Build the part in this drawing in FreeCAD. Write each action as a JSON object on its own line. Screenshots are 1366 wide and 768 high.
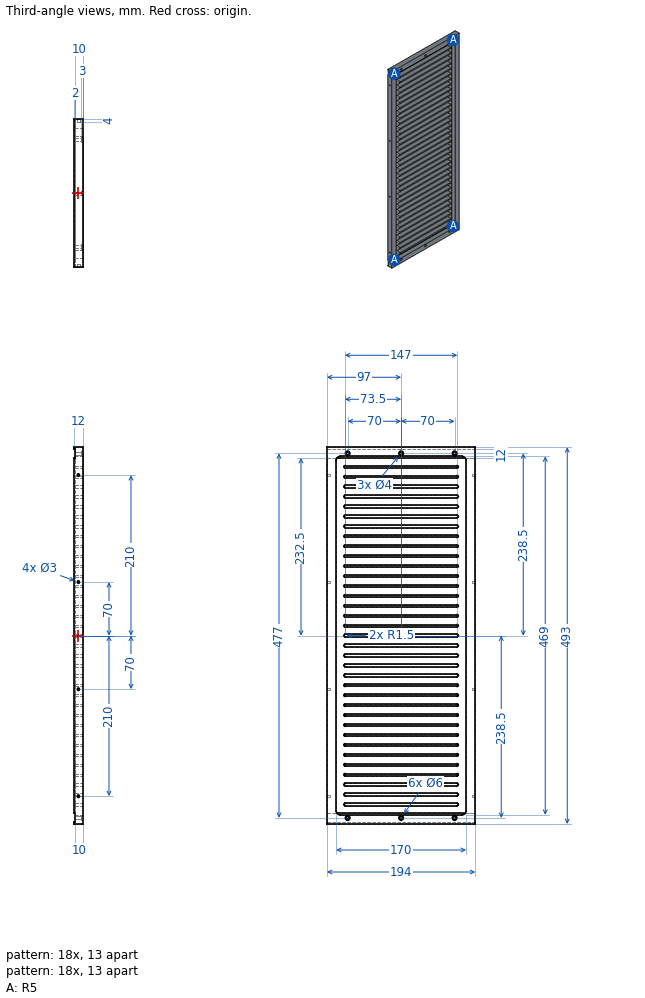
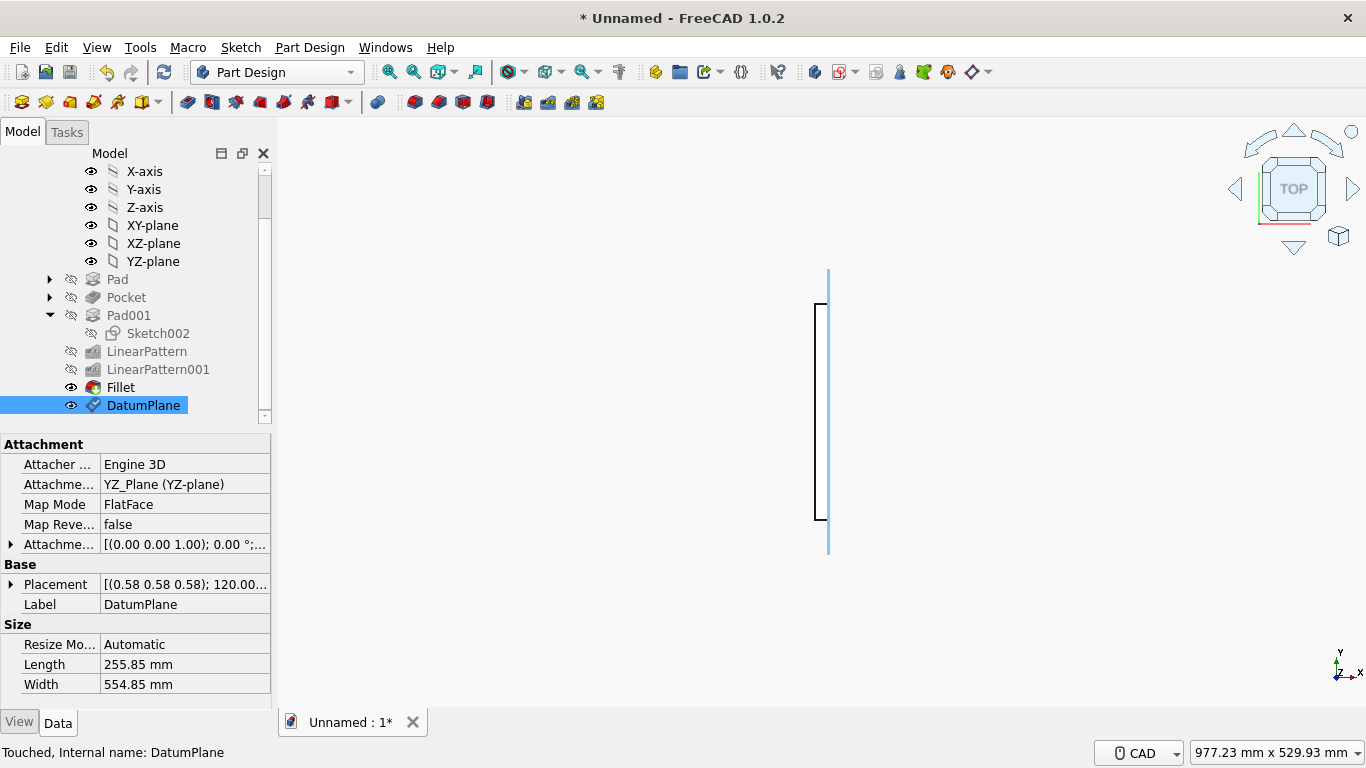
{"action": "left_click", "coordinate": [840, 72]}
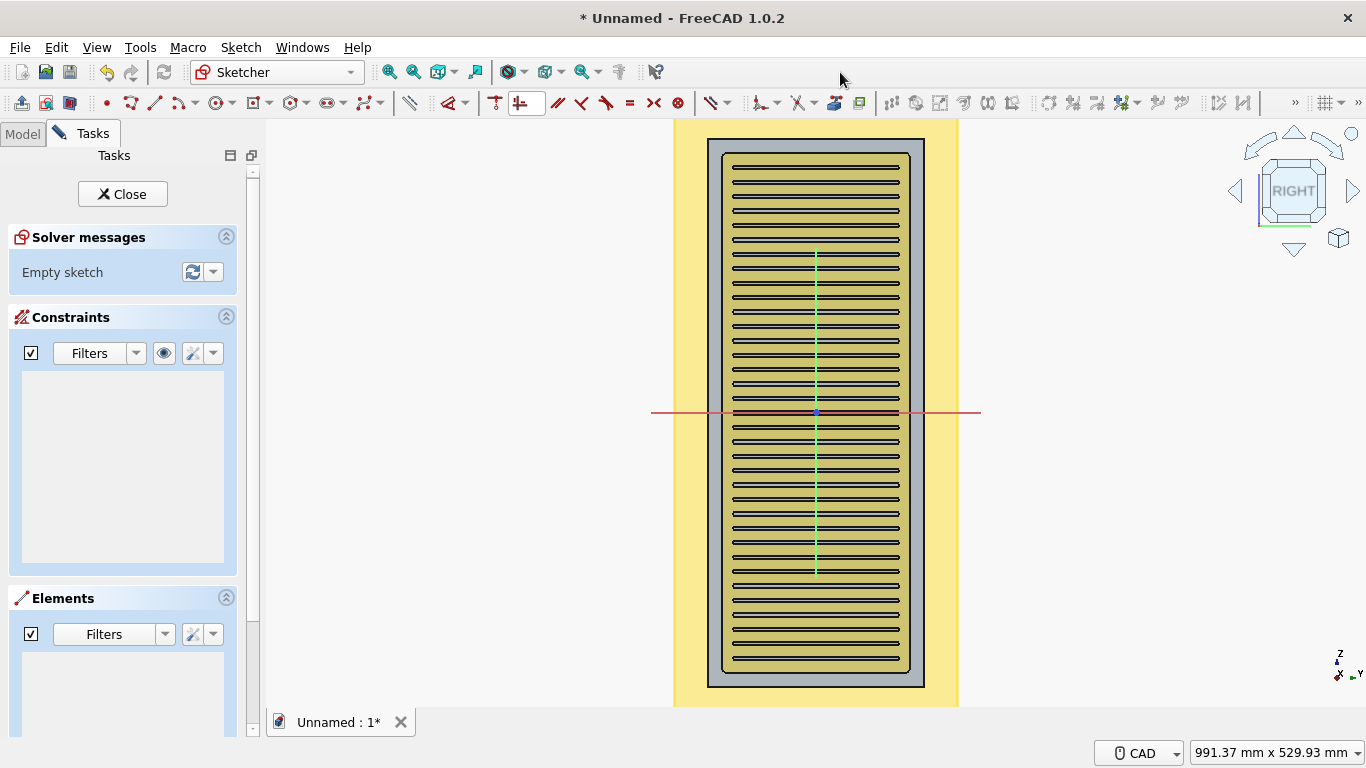
{"action": "scroll", "coordinate": [438, 679], "scroll_direction": "down", "scroll_amount": 1}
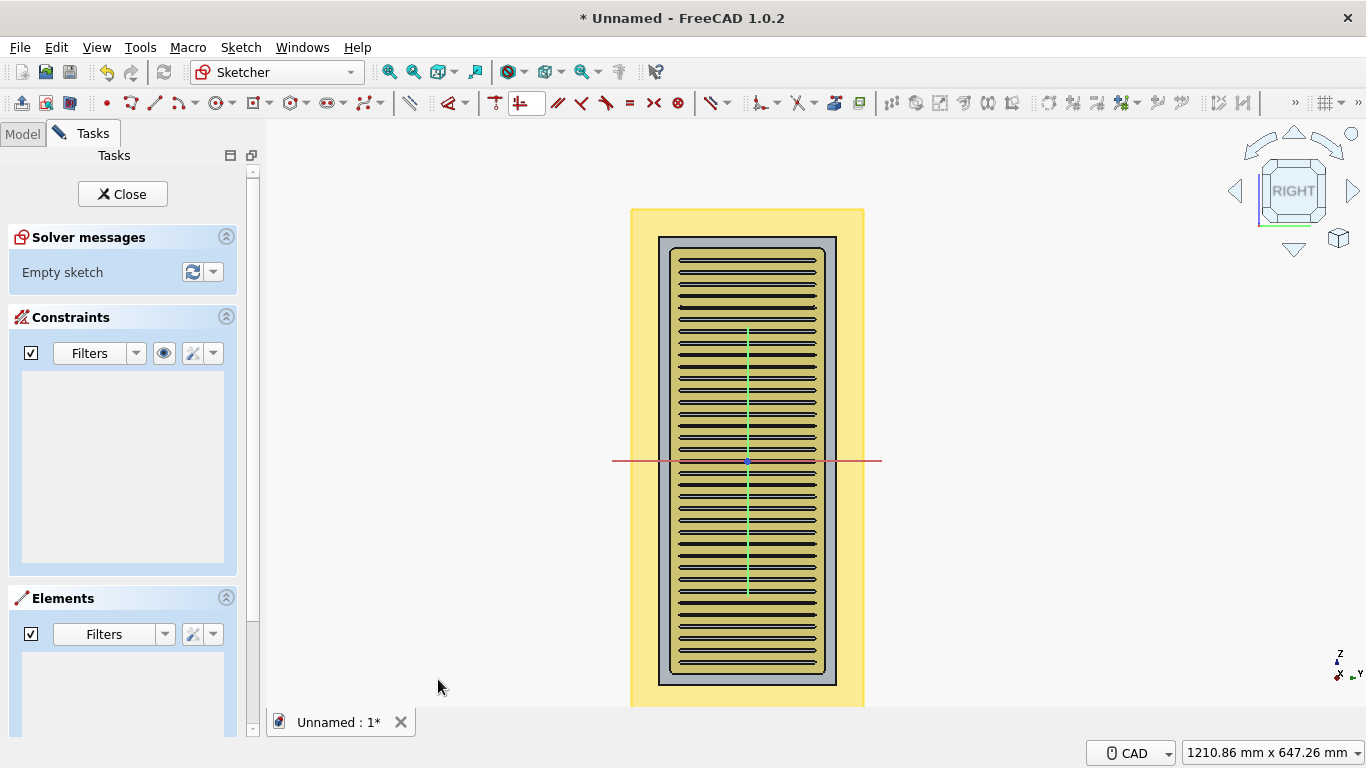
{"action": "scroll", "coordinate": [748, 278], "scroll_direction": "up", "scroll_amount": 3}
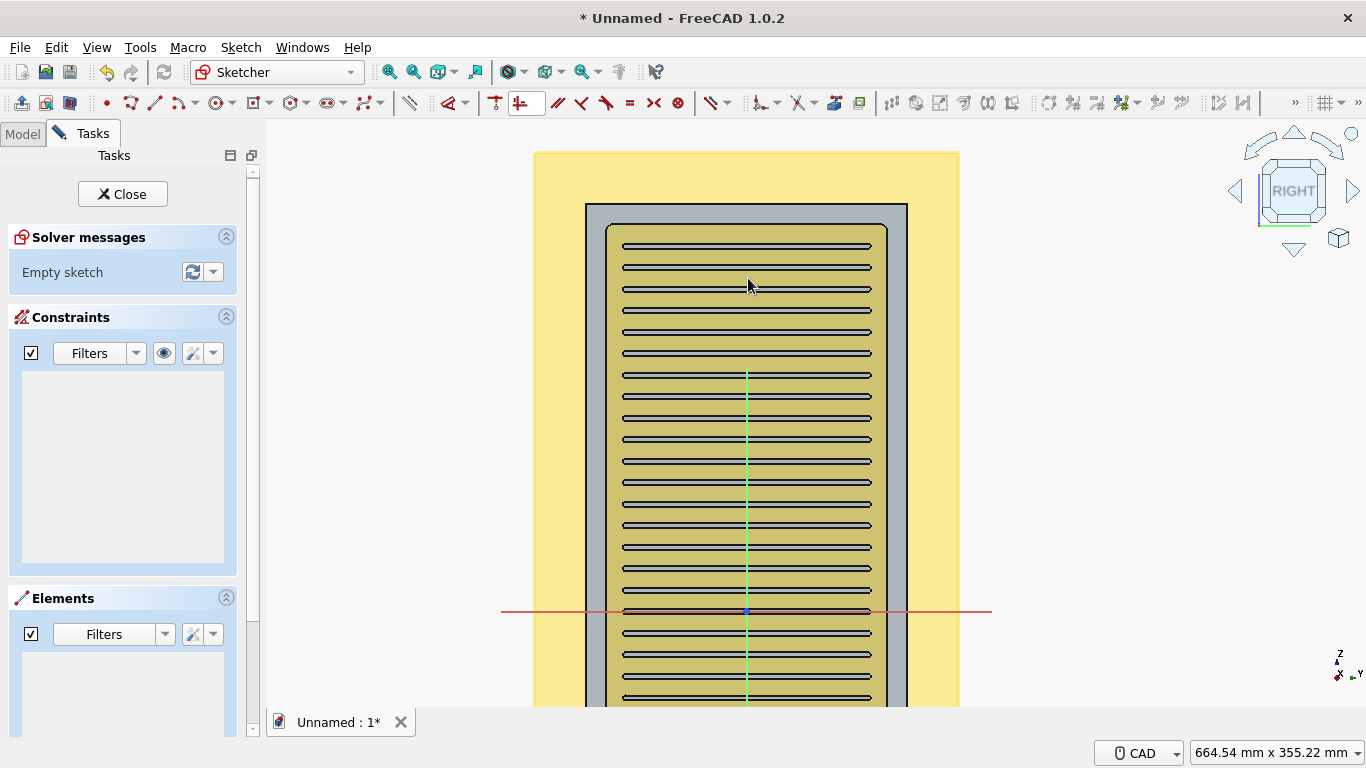
{"action": "left_click", "coordinate": [216, 104]}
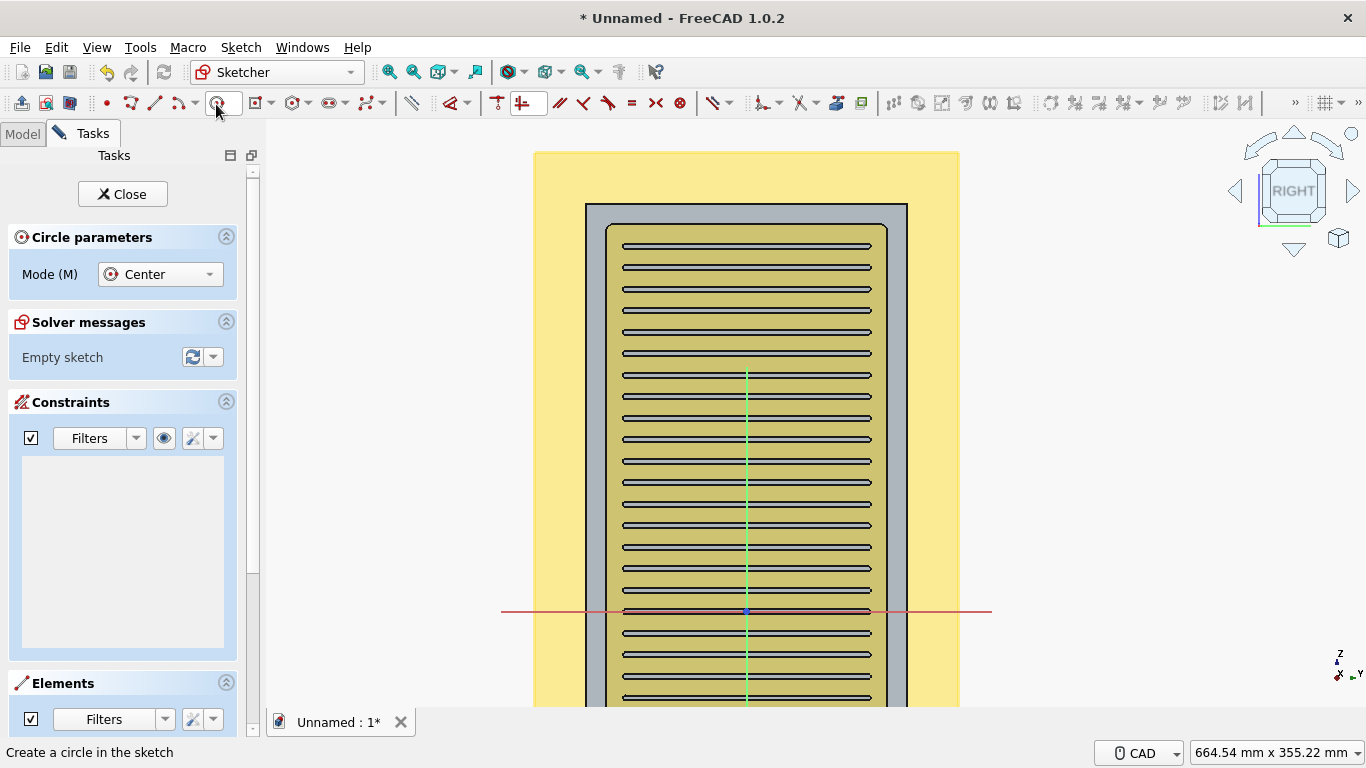
{"action": "scroll", "coordinate": [747, 217], "scroll_direction": "up", "scroll_amount": 10}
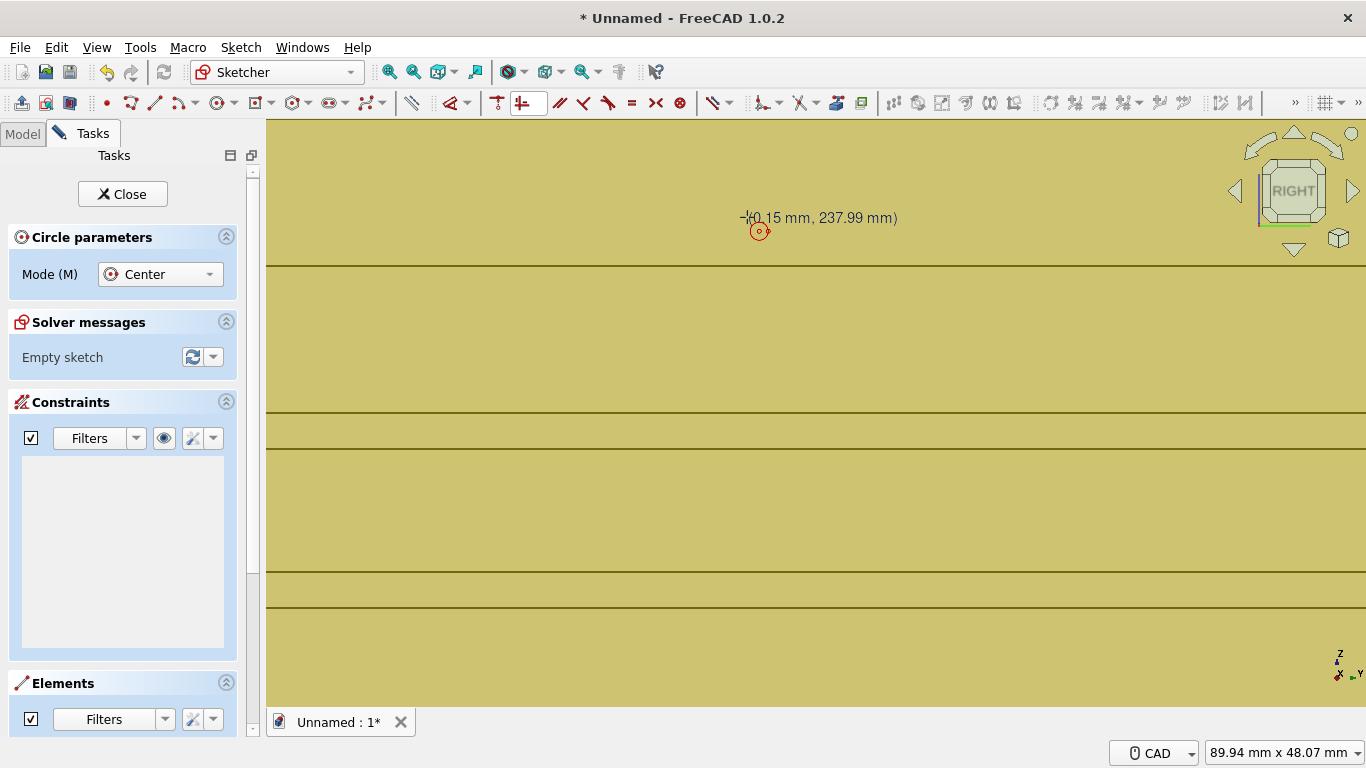
{"action": "scroll", "coordinate": [748, 217], "scroll_direction": "down", "scroll_amount": 10}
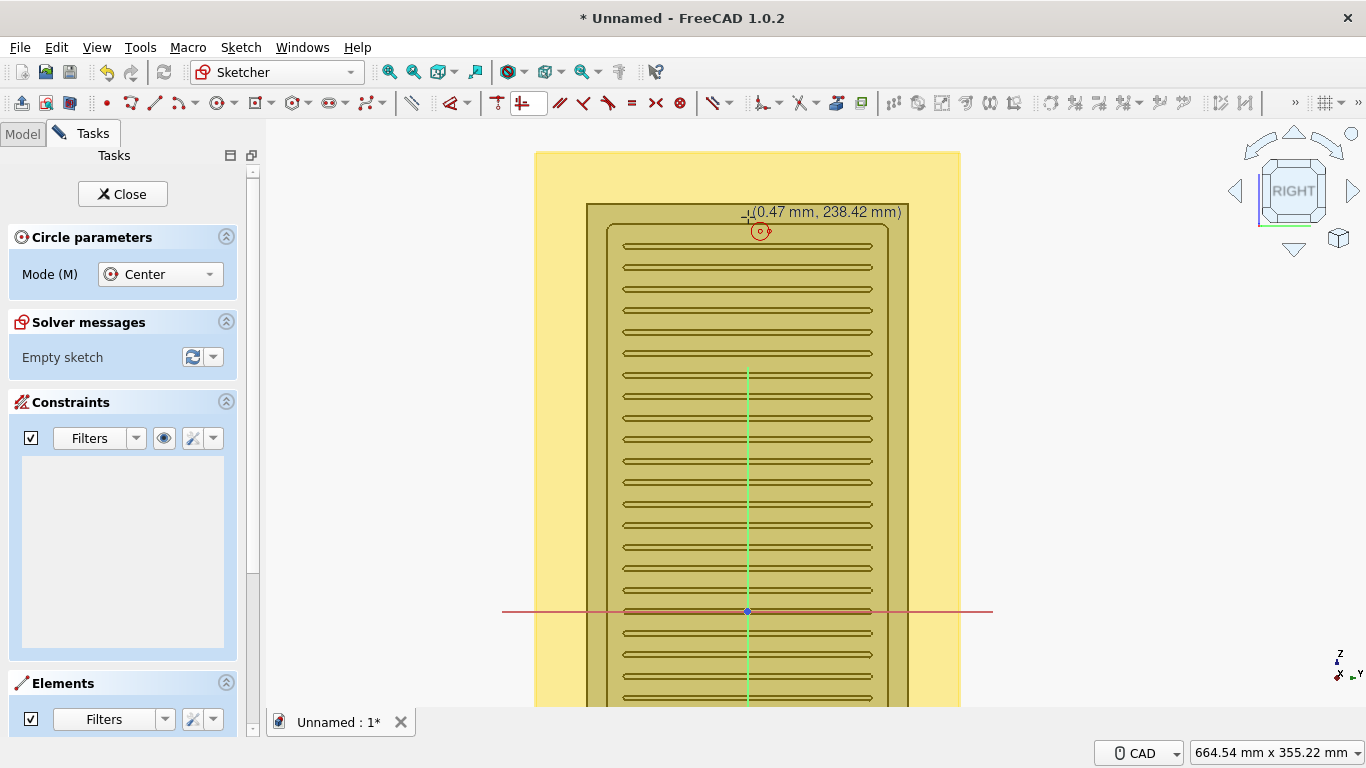
{"action": "left_click", "coordinate": [748, 217]}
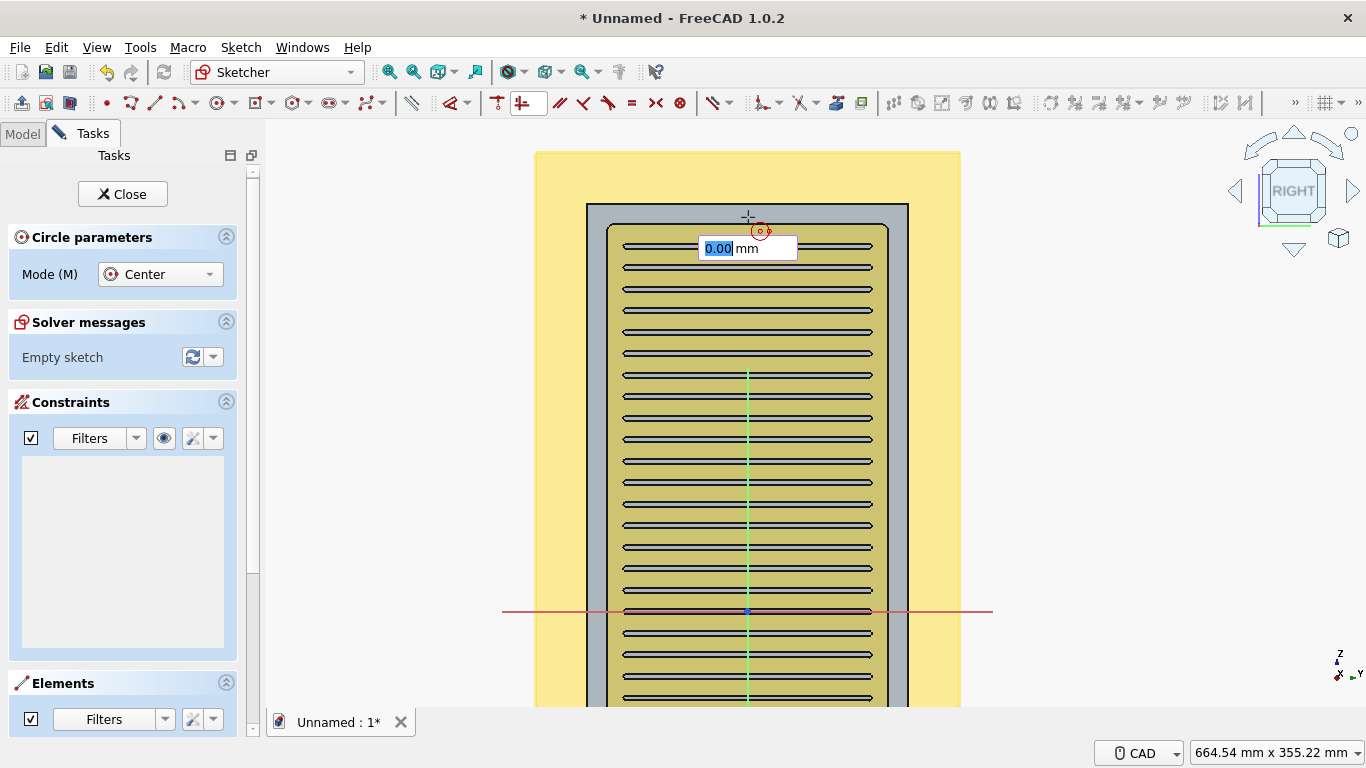
{"action": "scroll", "coordinate": [751, 216], "scroll_direction": "up", "scroll_amount": 9}
{"action": "mouse_move", "coordinate": [747, 215]}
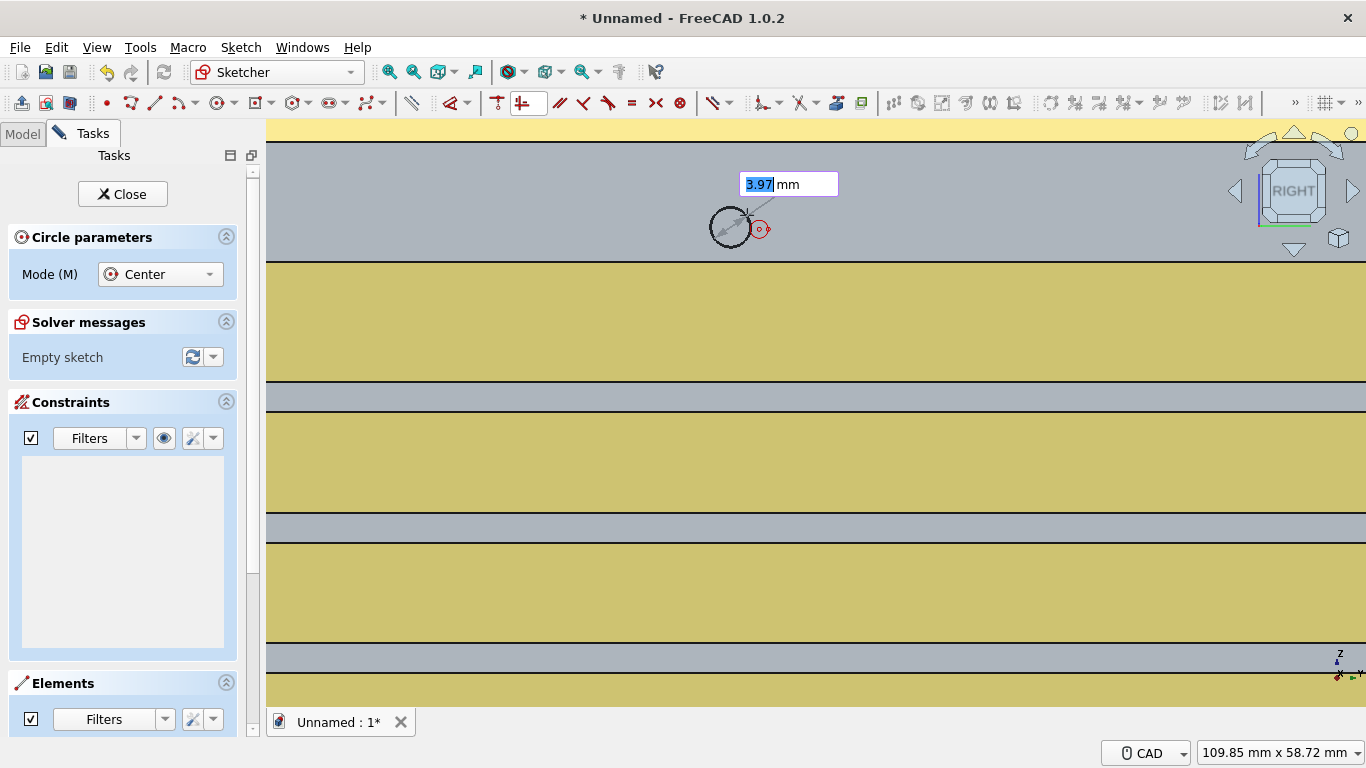
{"action": "type", "text": "4"}
{"action": "key", "text": "Return"}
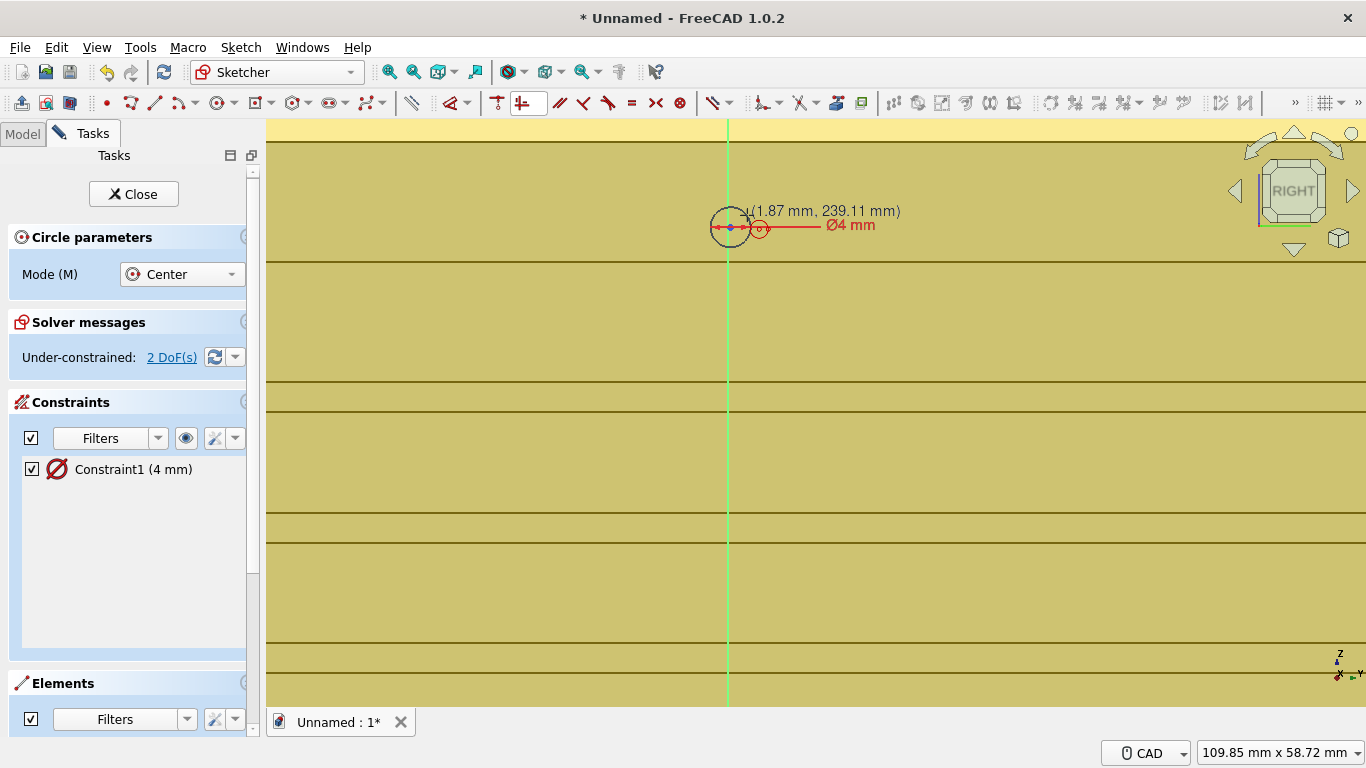
{"action": "scroll", "coordinate": [751, 216], "scroll_direction": "down", "scroll_amount": 9}